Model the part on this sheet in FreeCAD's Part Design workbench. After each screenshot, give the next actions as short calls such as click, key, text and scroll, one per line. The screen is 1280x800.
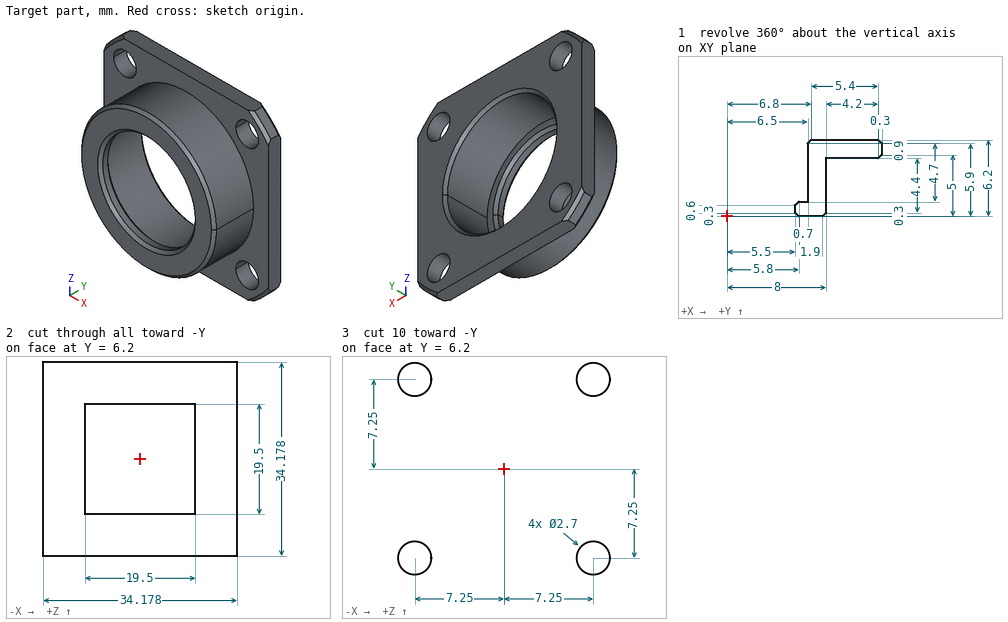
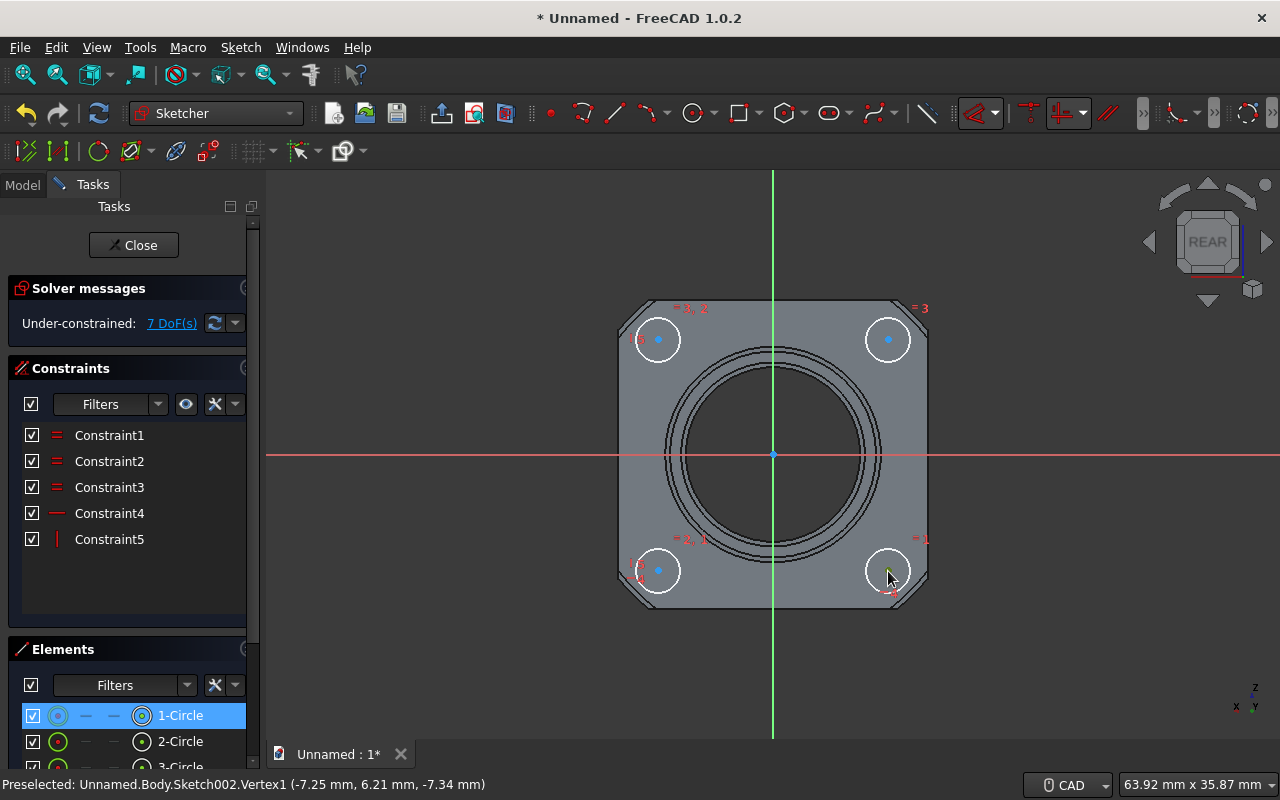
click(888, 340)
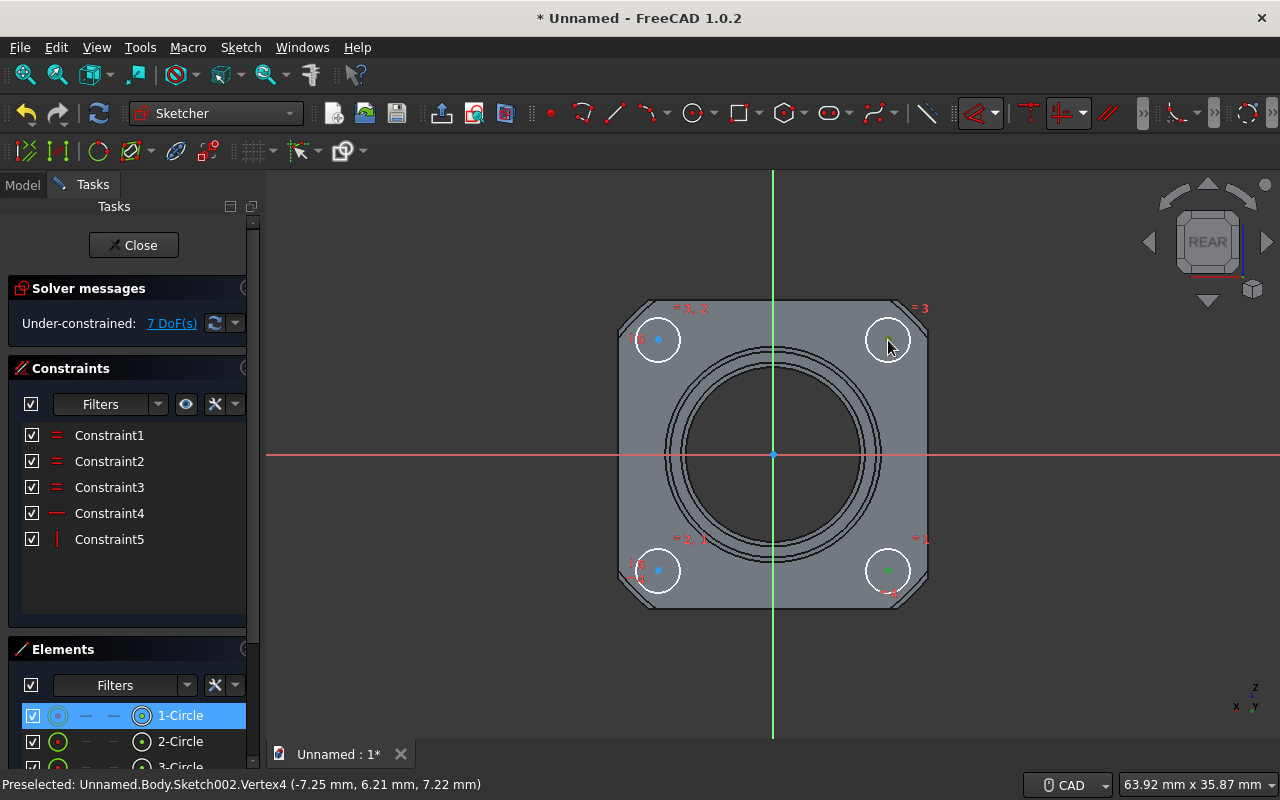
click(1086, 114)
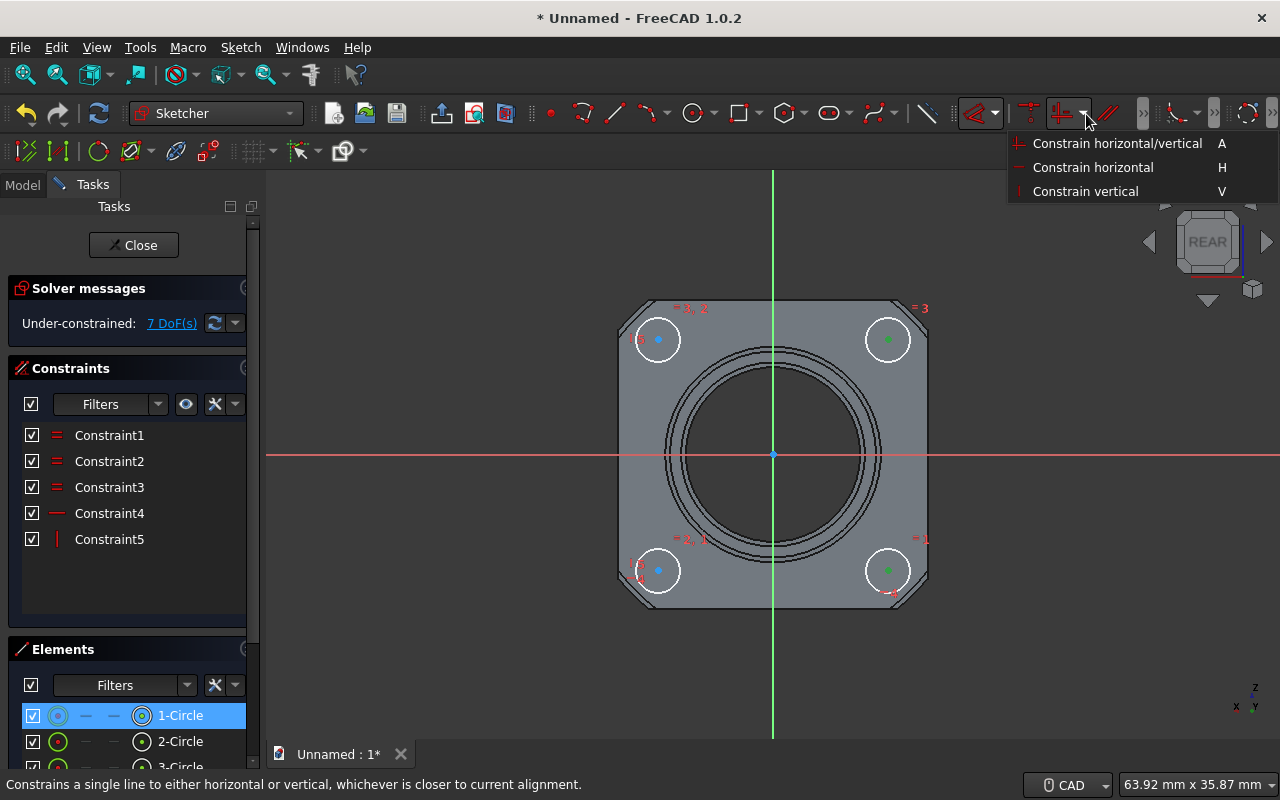
click(1143, 191)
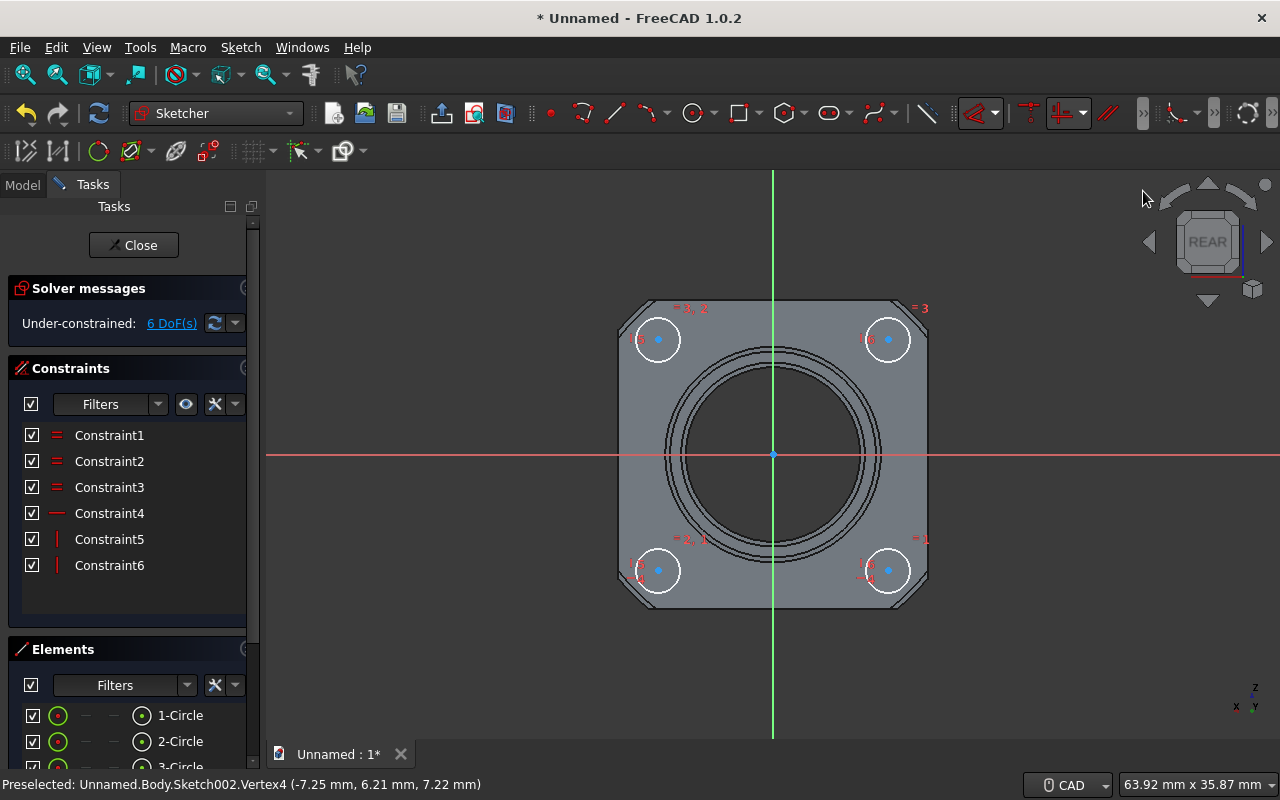
click(658, 340)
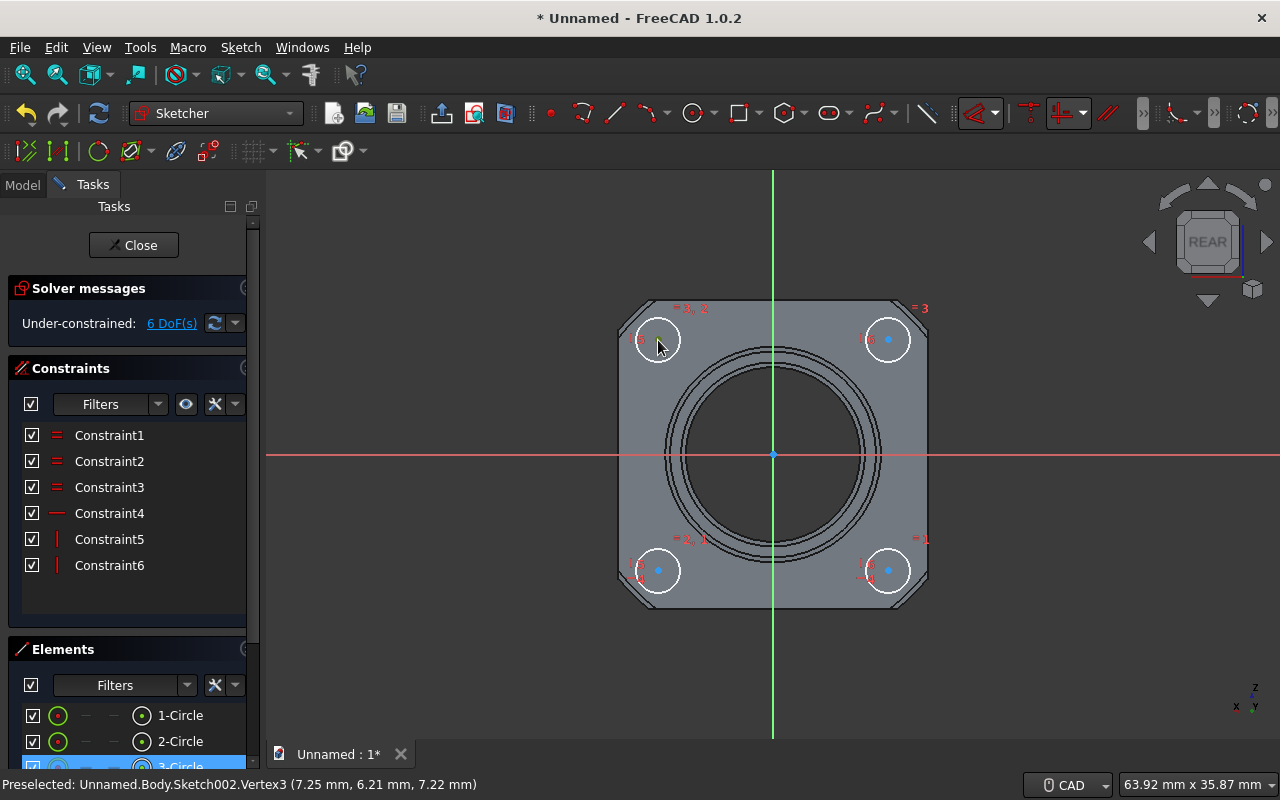
click(888, 340)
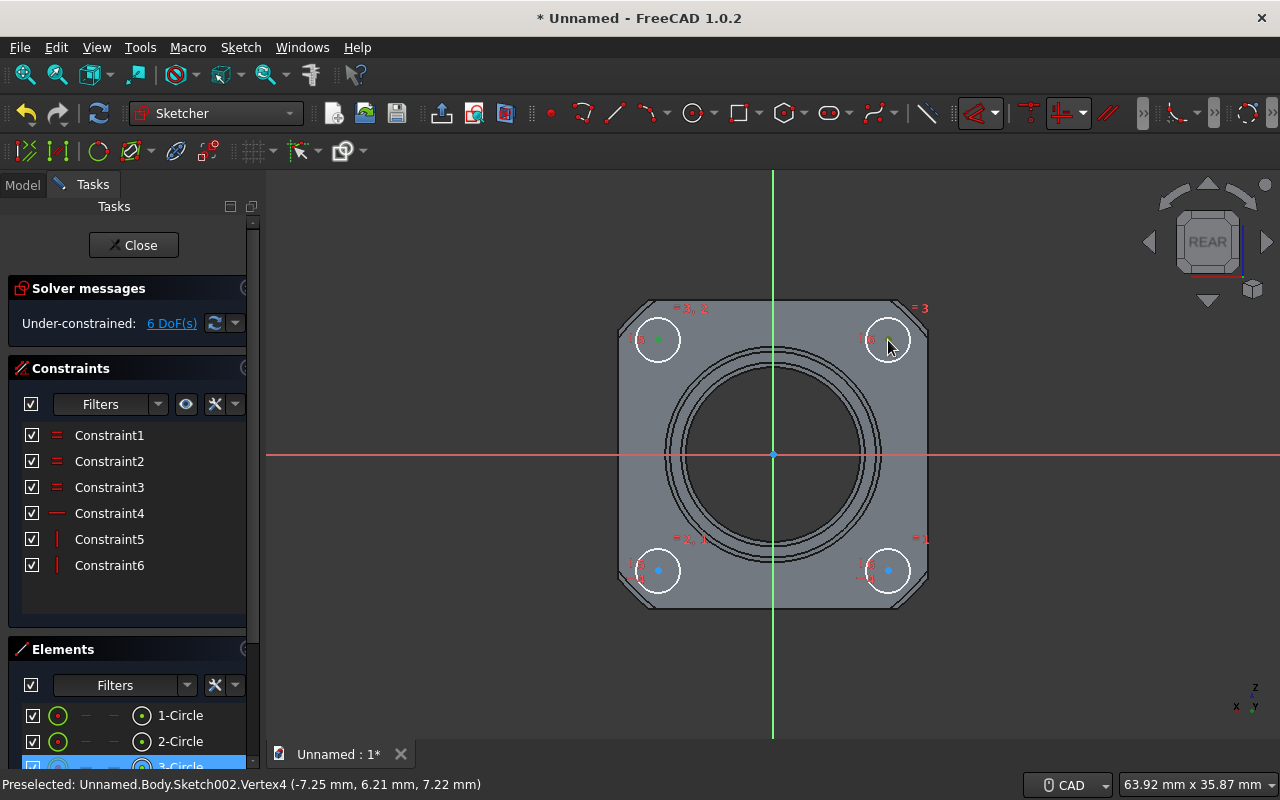
key(h)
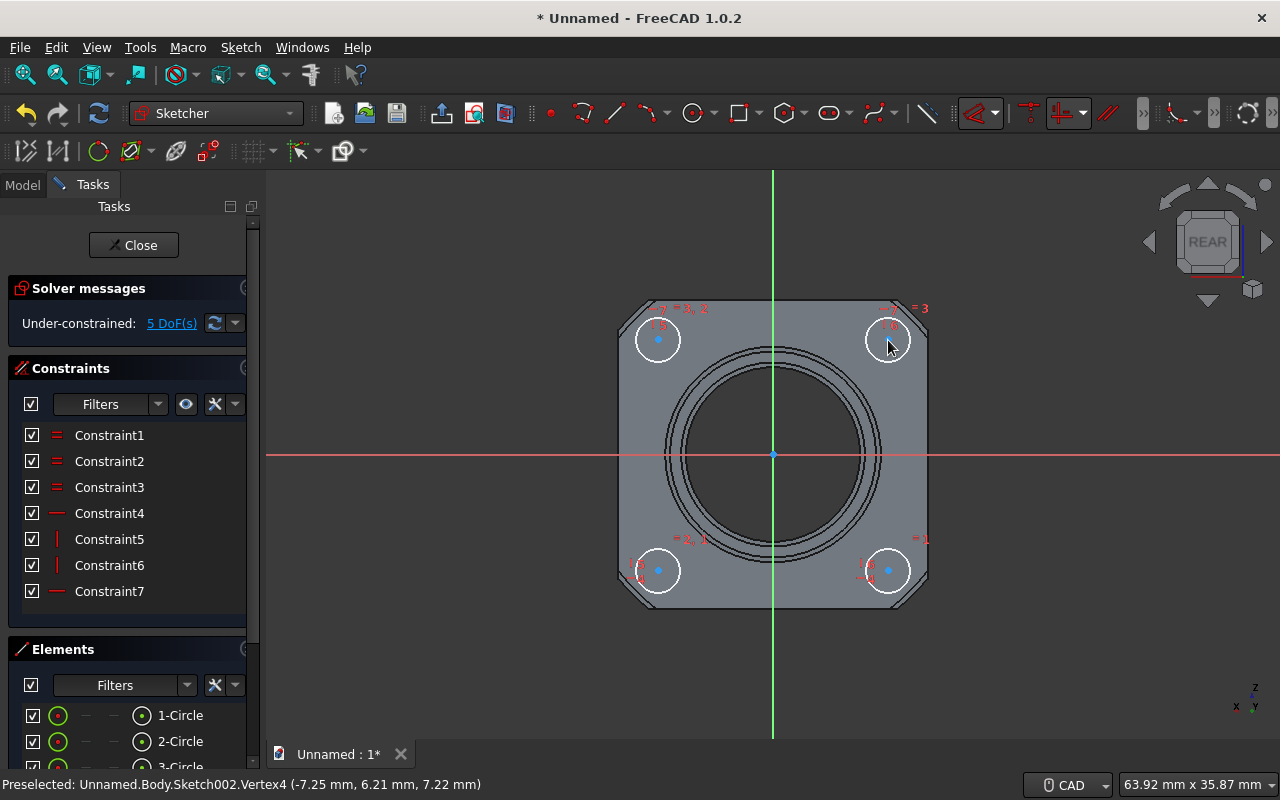
click(903, 555)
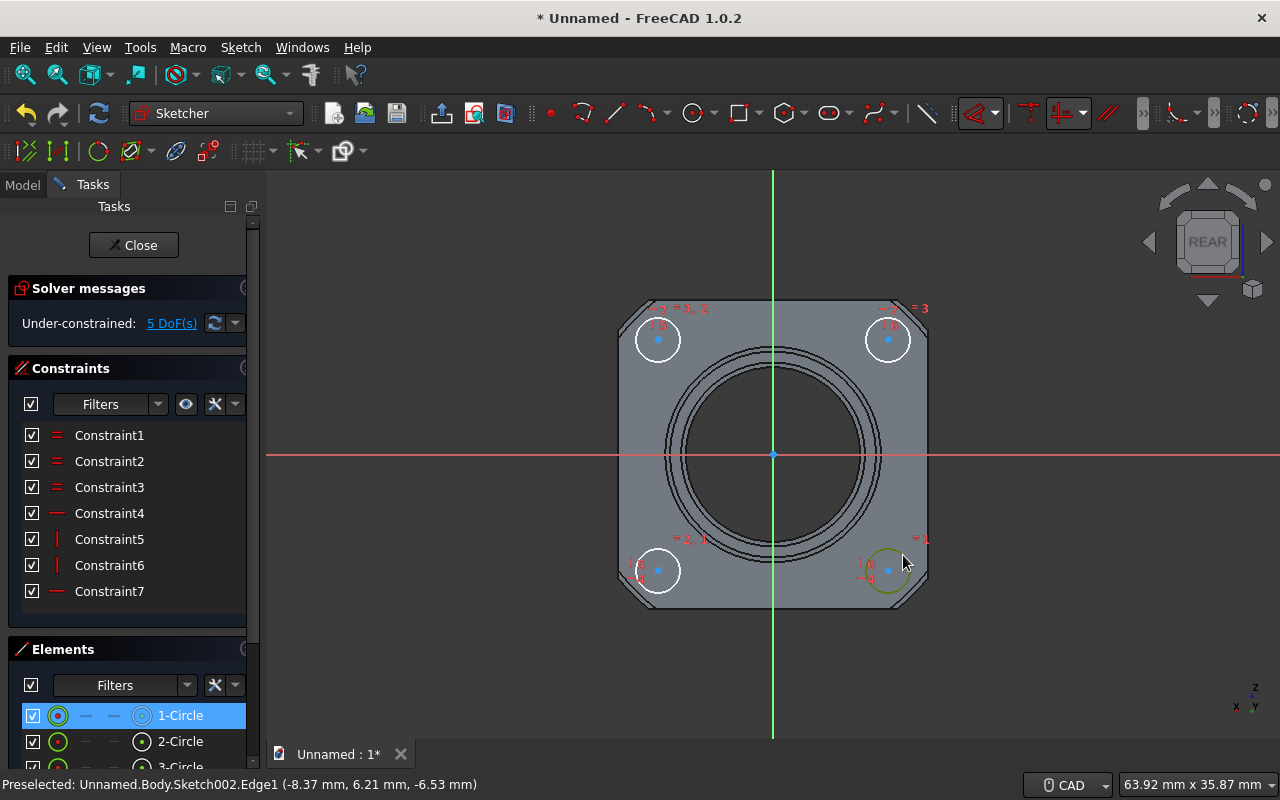
key(k)
key(o)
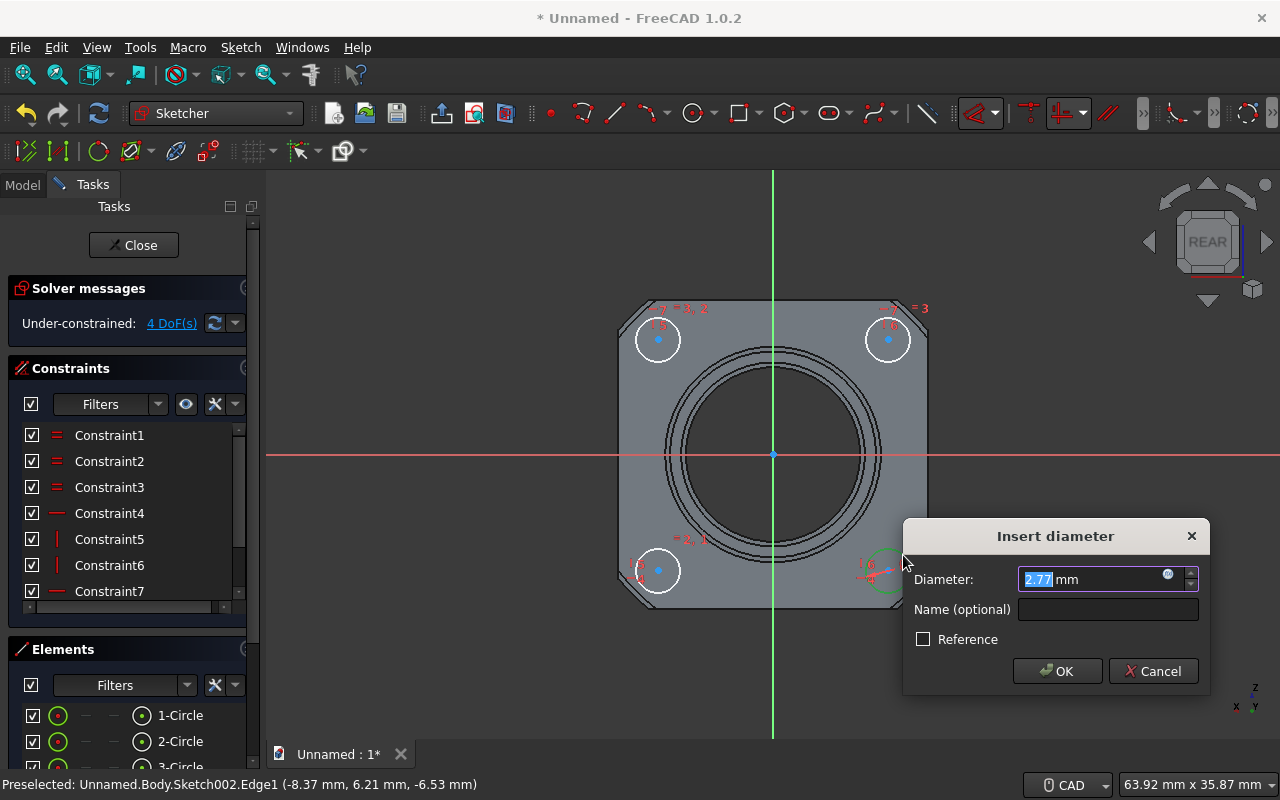
text(2.7)
key(Return)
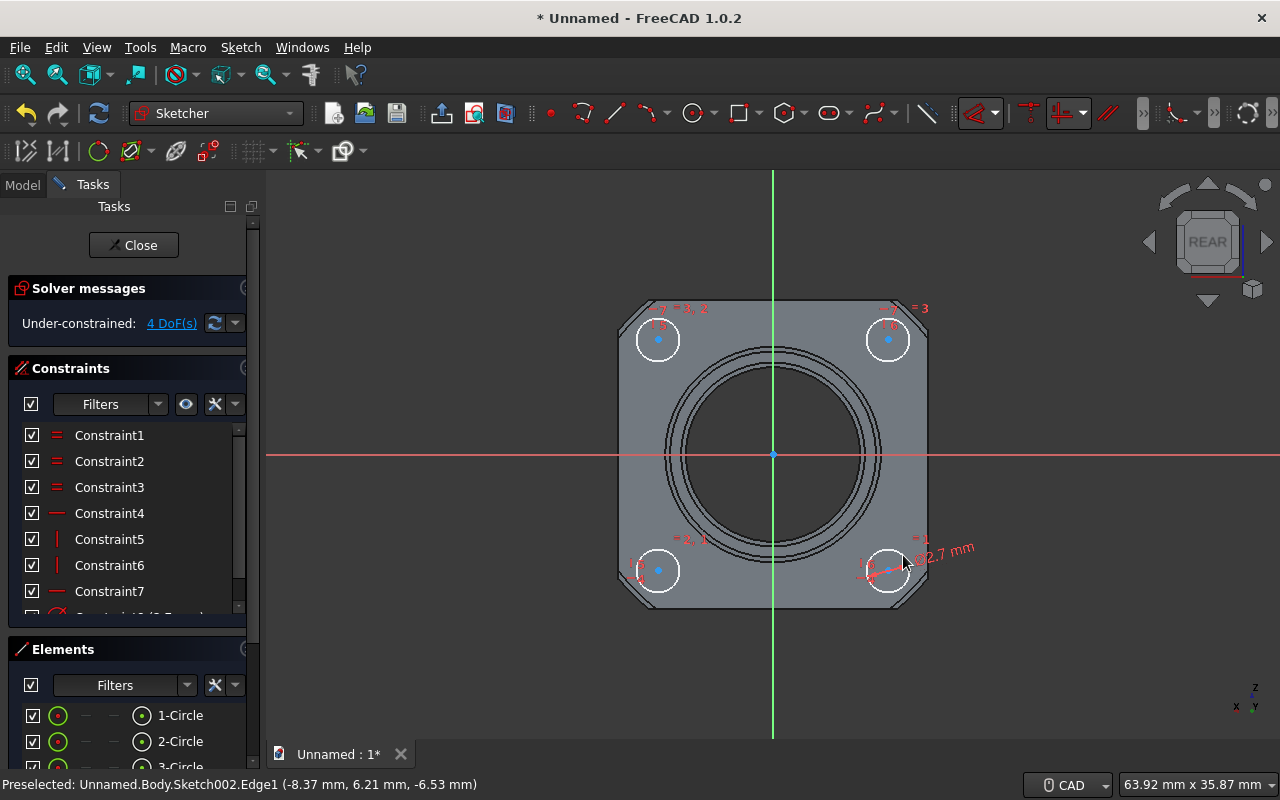
click(888, 571)